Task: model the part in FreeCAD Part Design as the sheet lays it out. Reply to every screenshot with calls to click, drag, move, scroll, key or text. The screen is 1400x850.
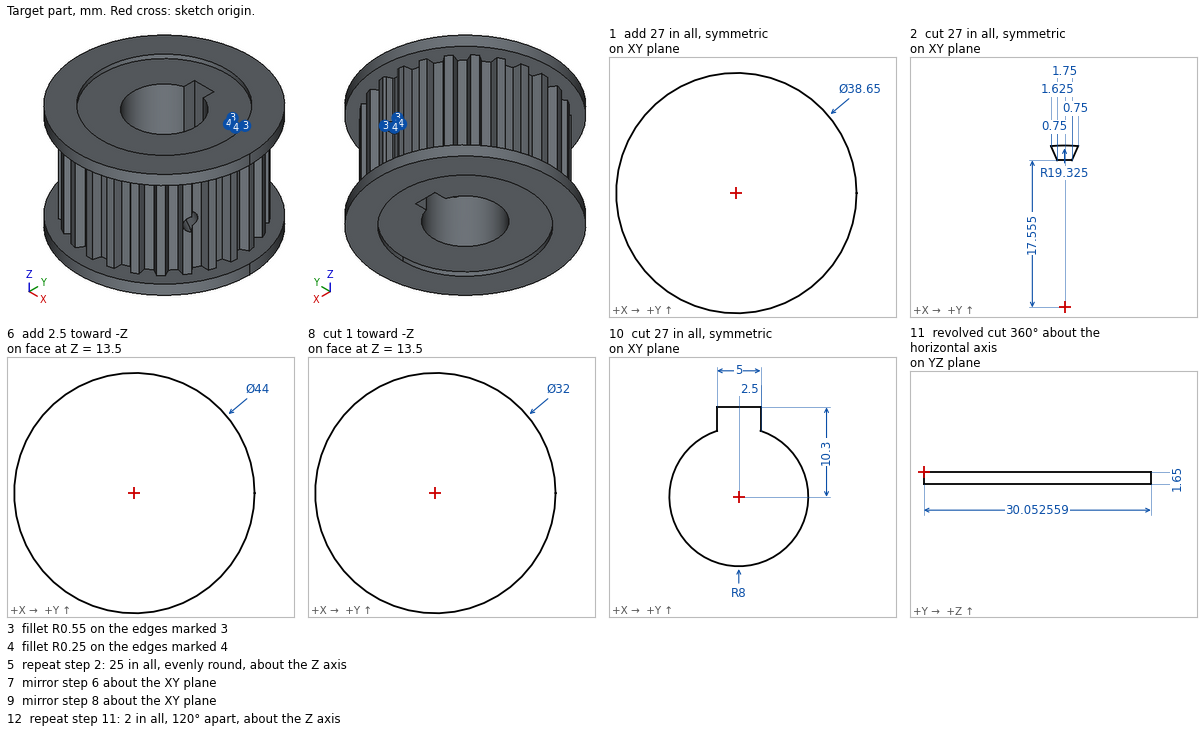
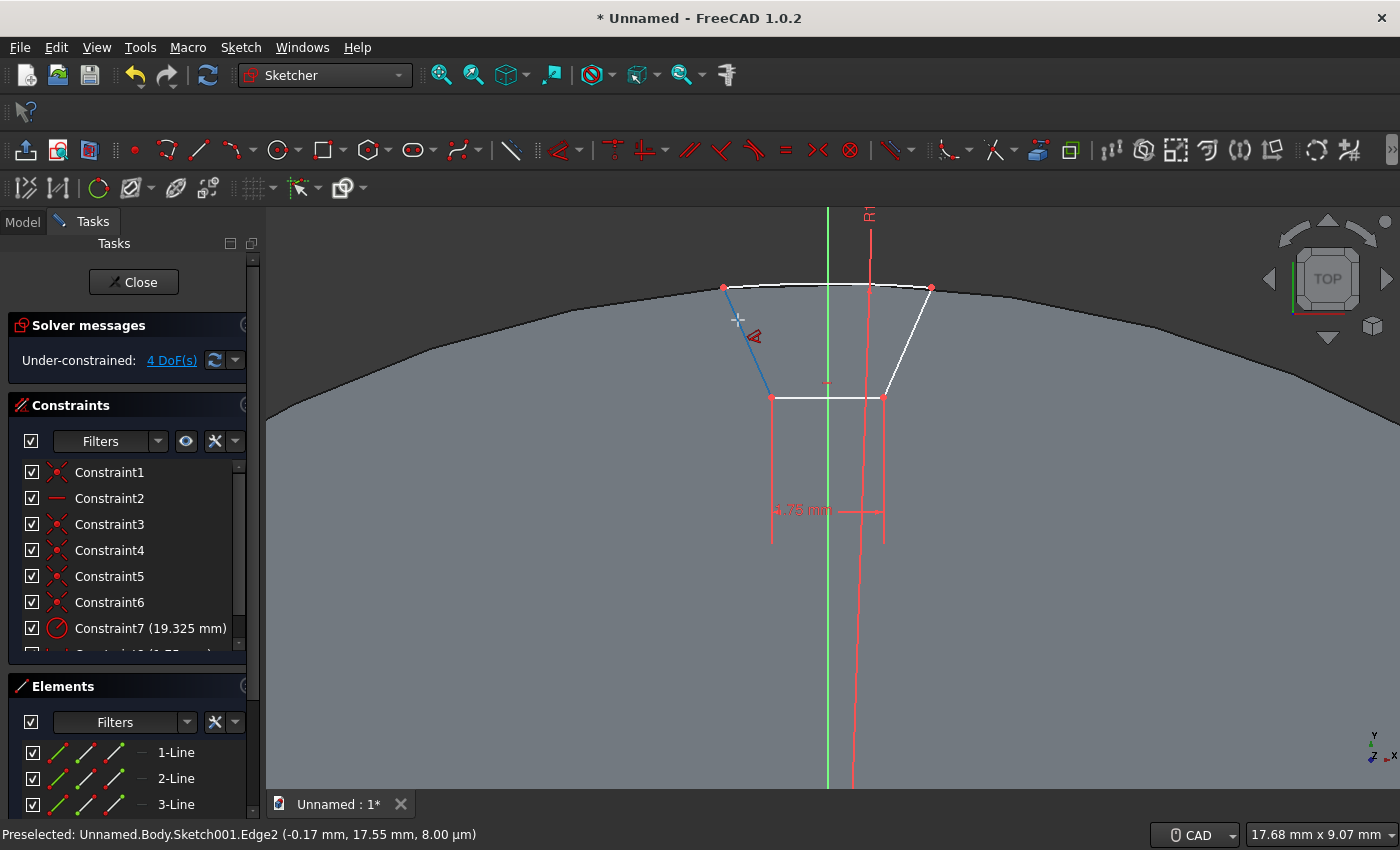
click(738, 321)
click(748, 432)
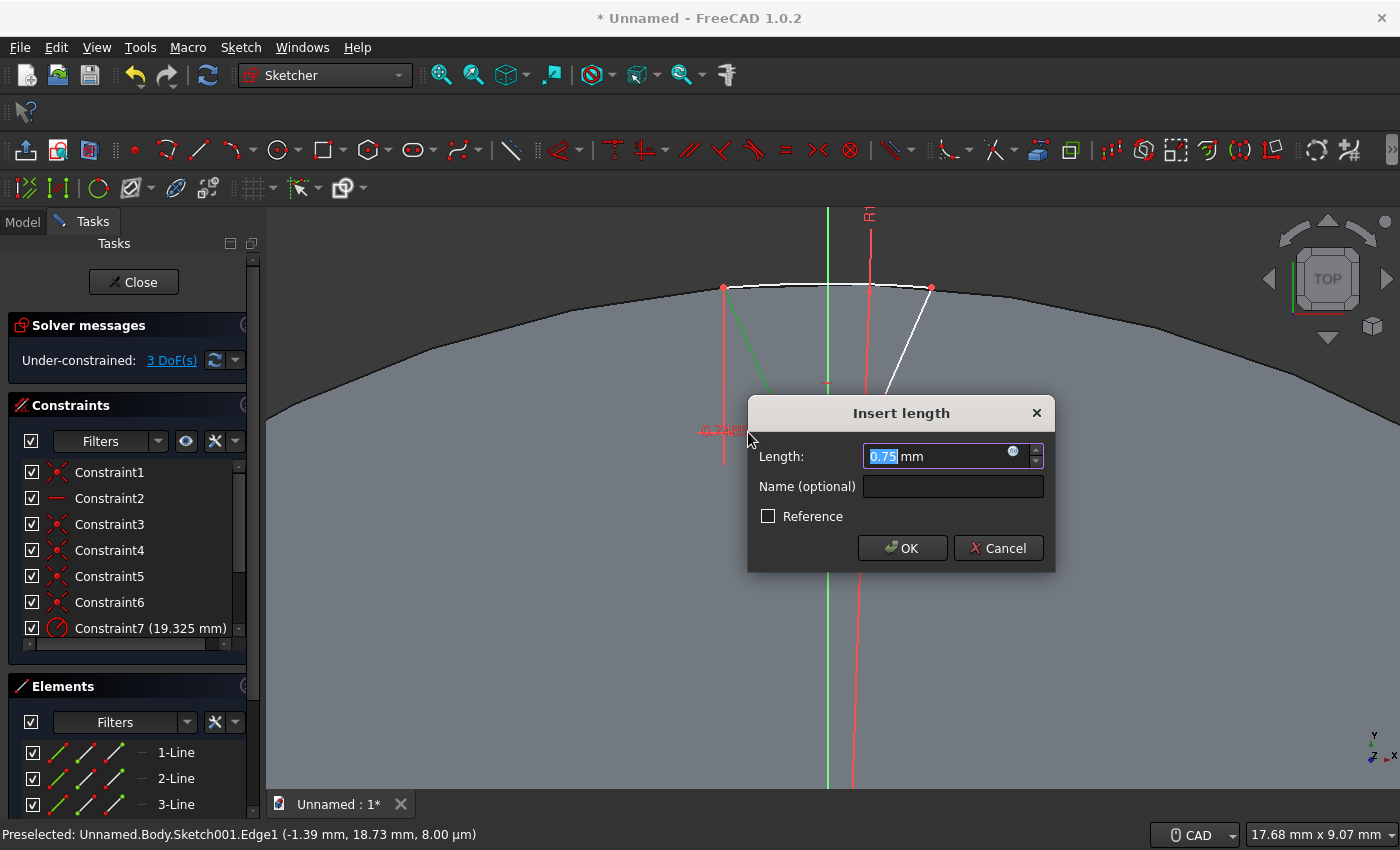
text(0.75)
key(Return)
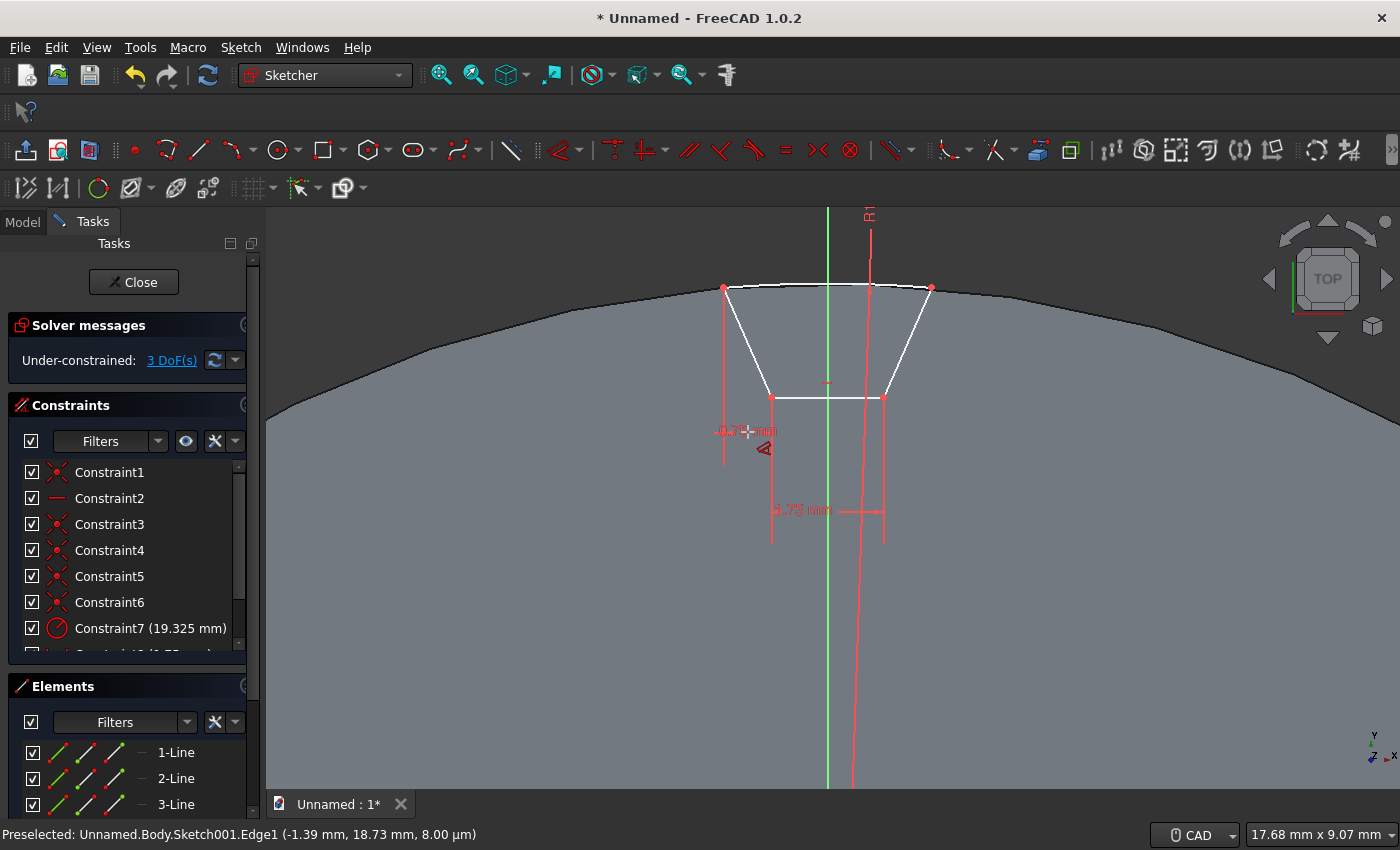
click(898, 365)
click(908, 432)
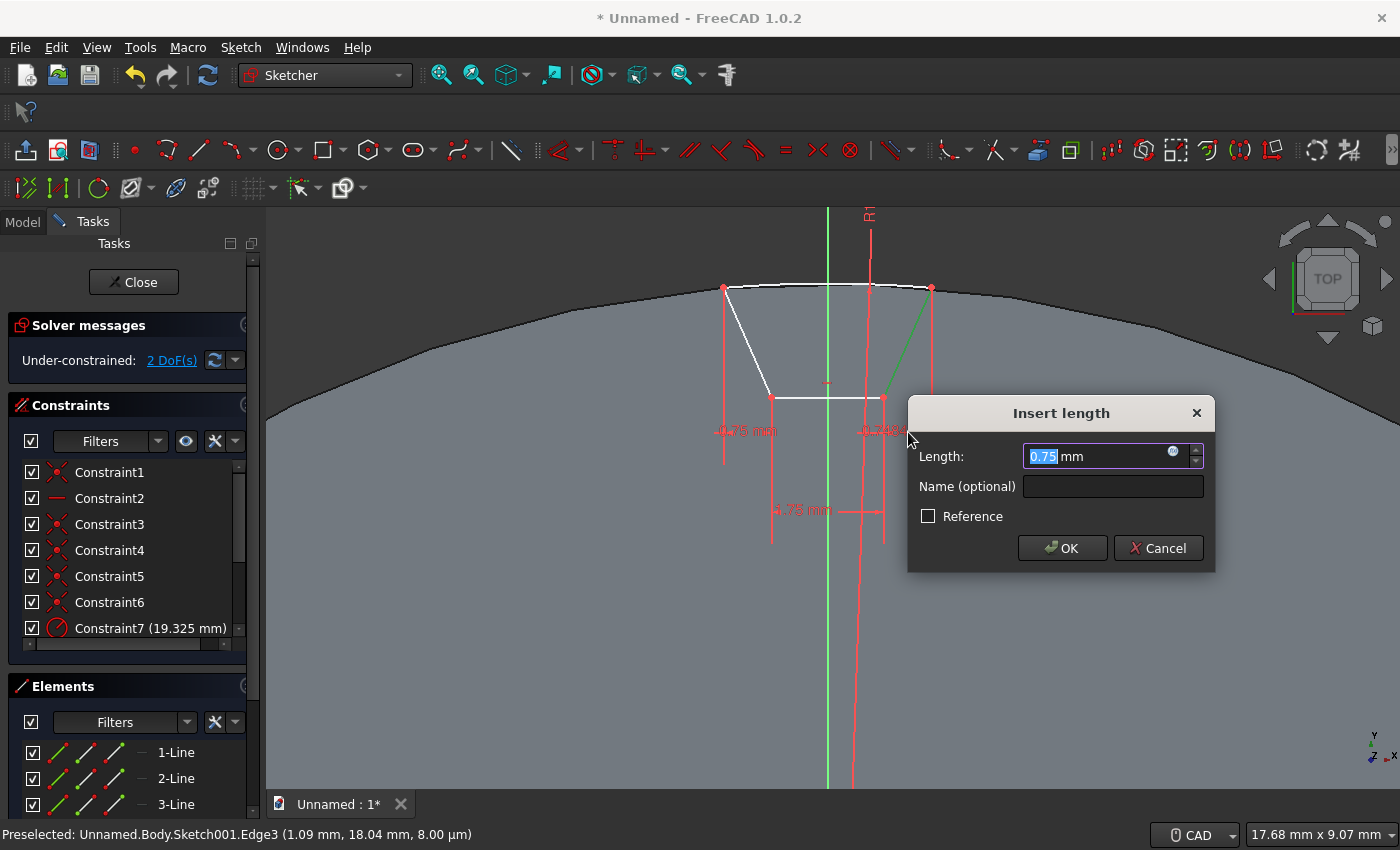
text(0.75)
key(Return)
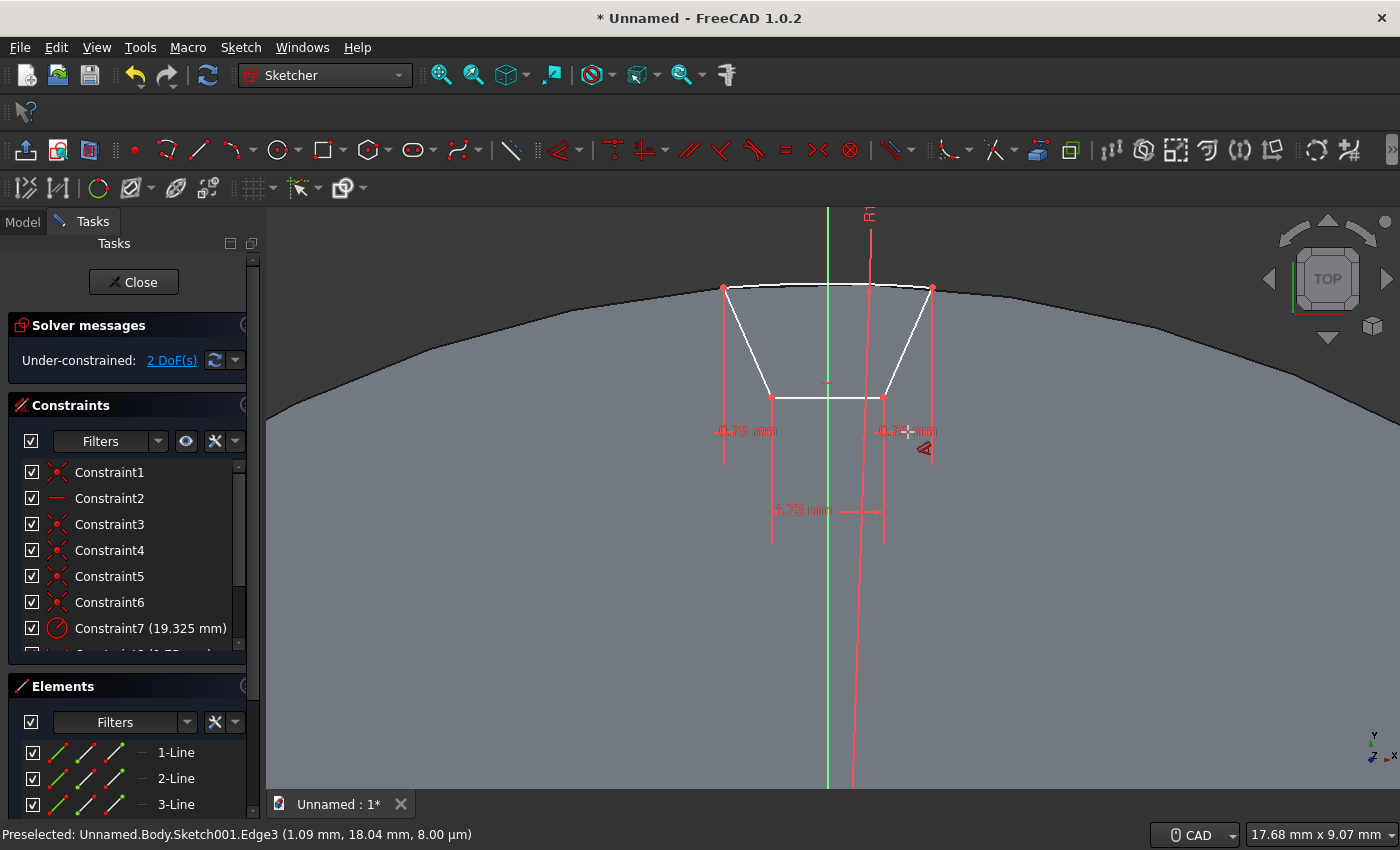
click(724, 288)
click(776, 254)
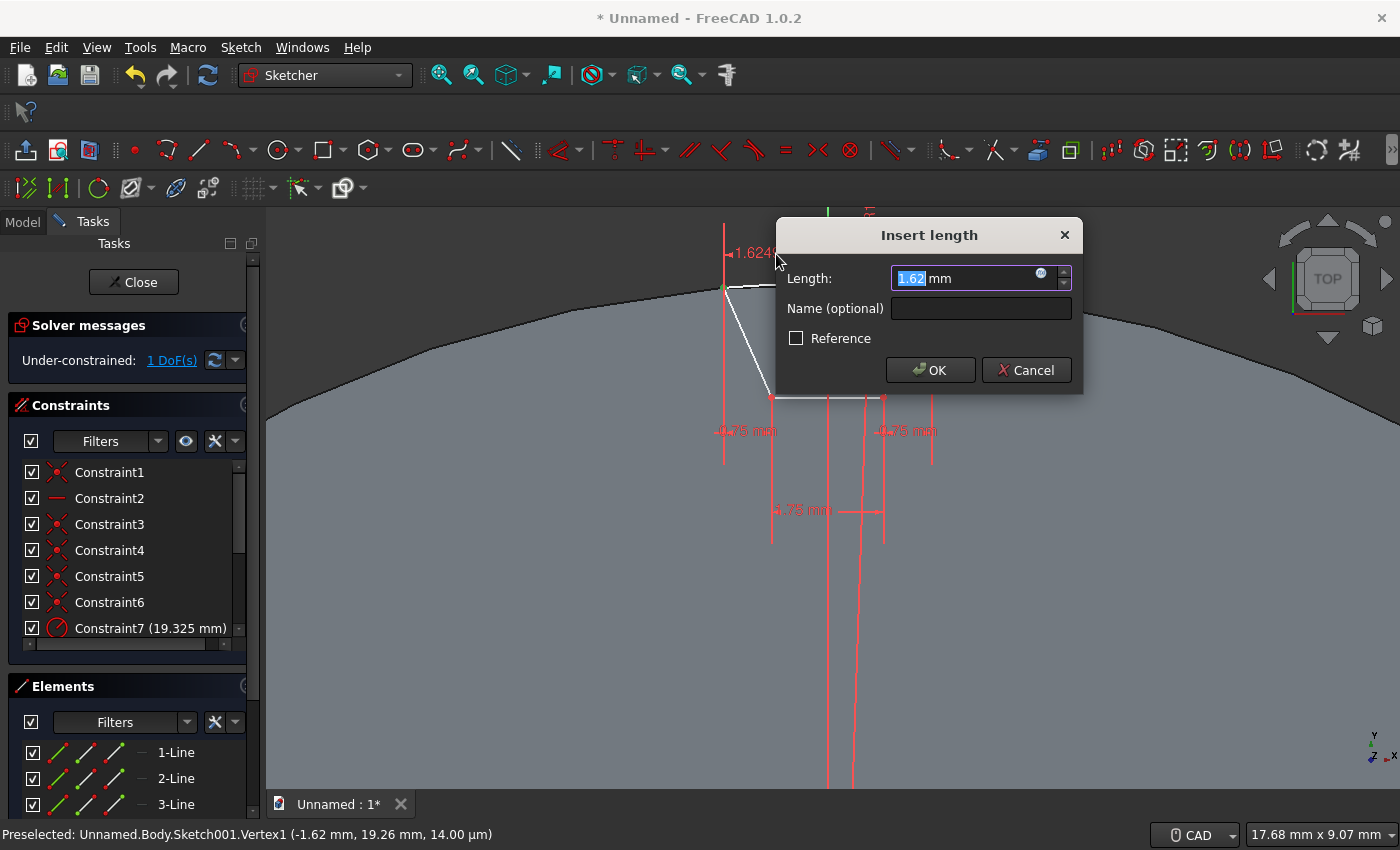
text(1.625)
key(Return)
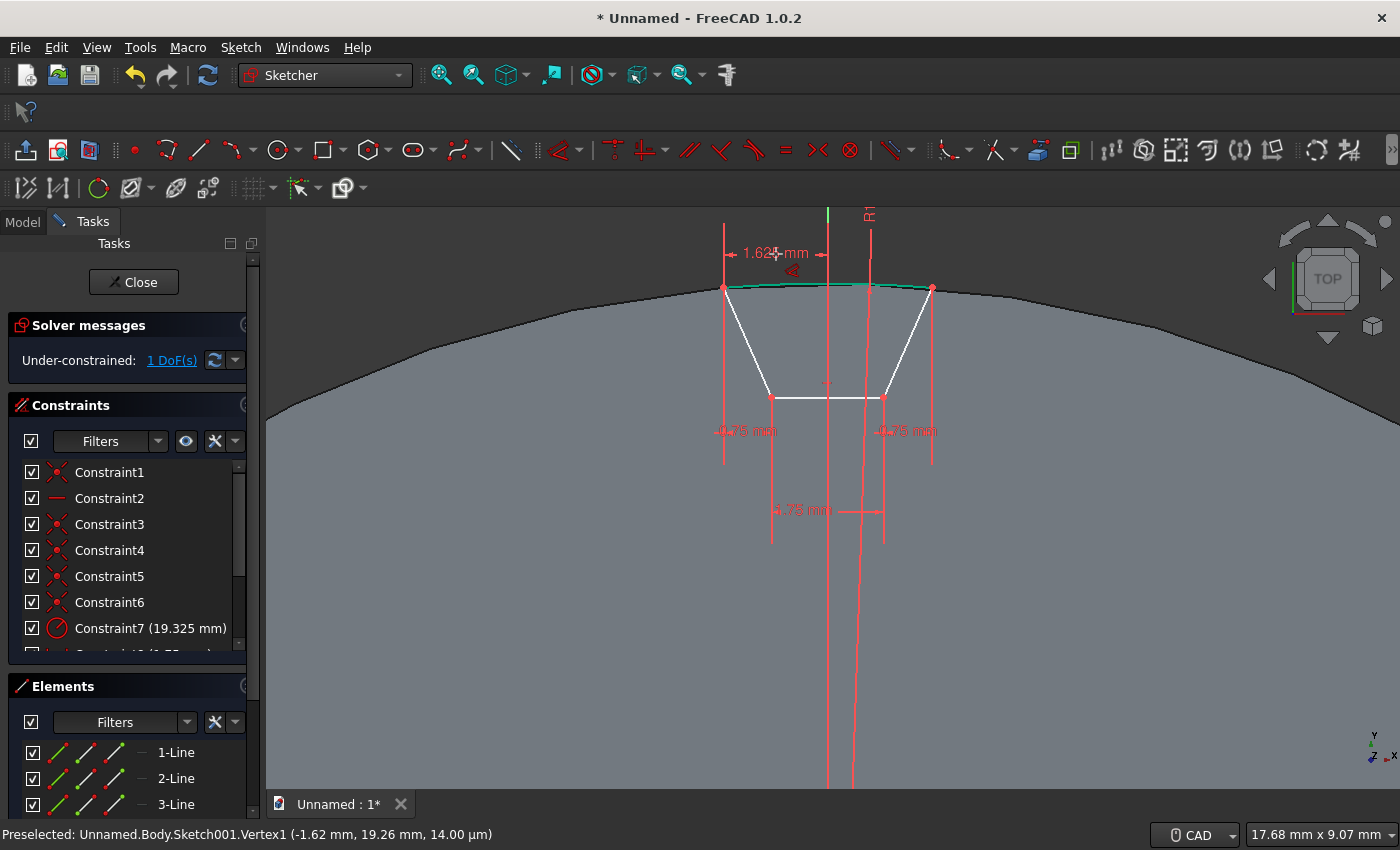
click(772, 398)
click(738, 579)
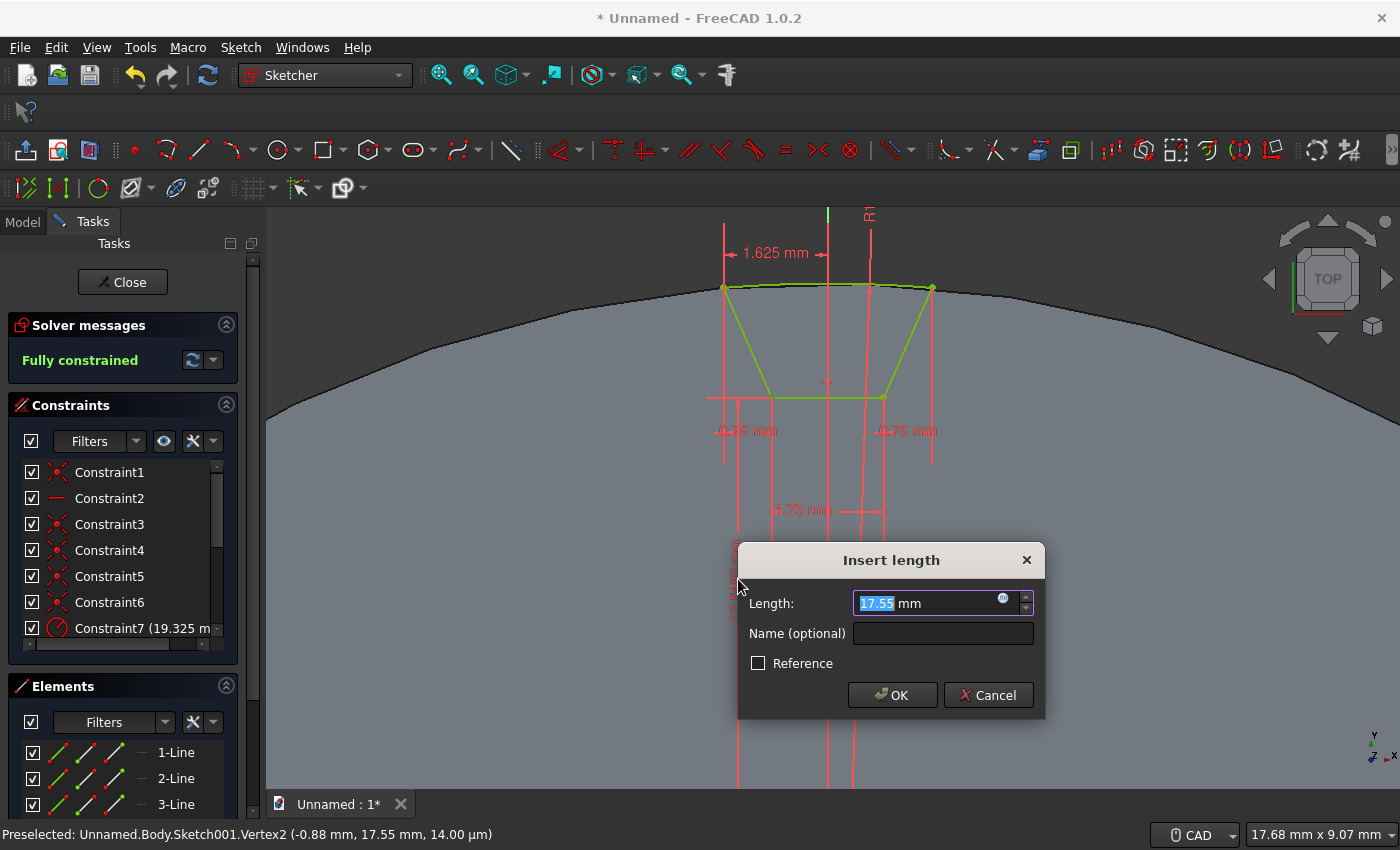
text(17.555)
key(Return)
key(Escape)